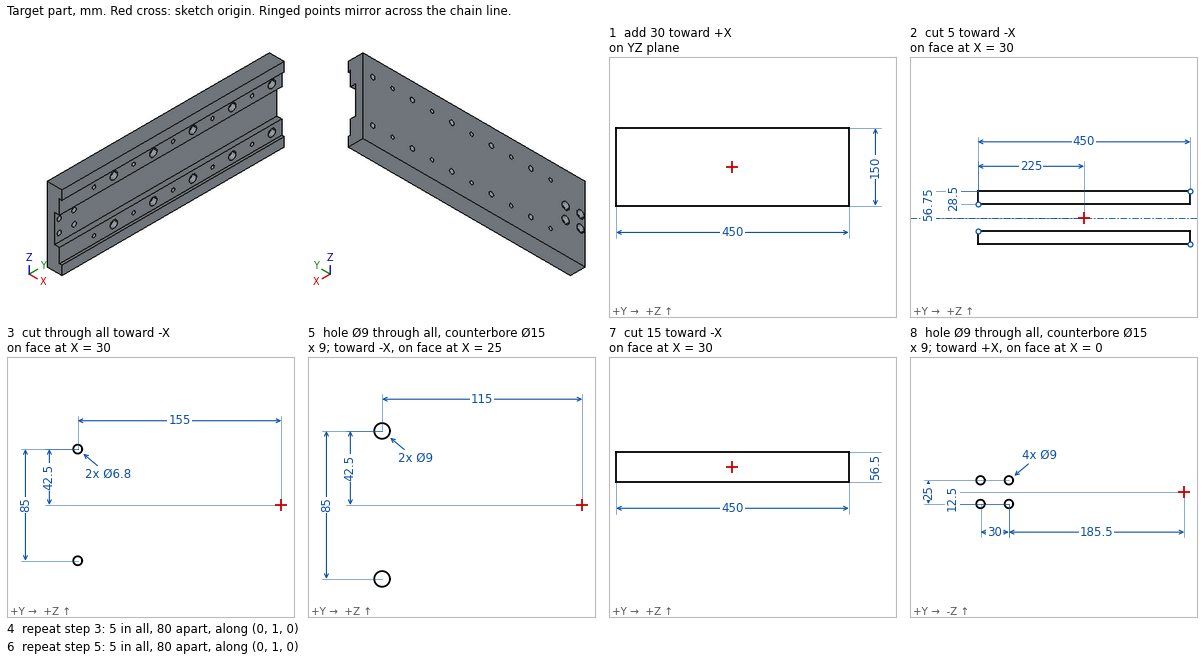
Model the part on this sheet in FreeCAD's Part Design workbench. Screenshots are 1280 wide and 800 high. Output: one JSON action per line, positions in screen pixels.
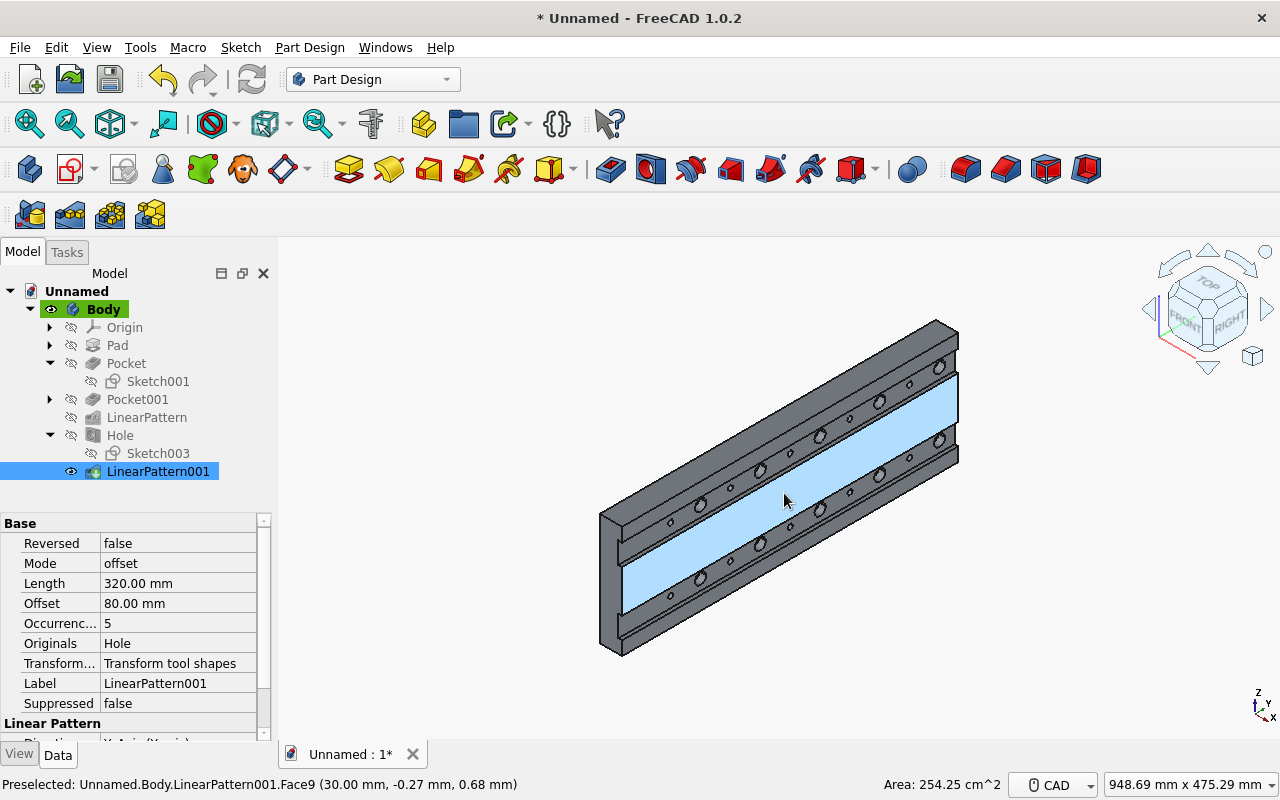
{"action": "left_click", "coordinate": [70, 170]}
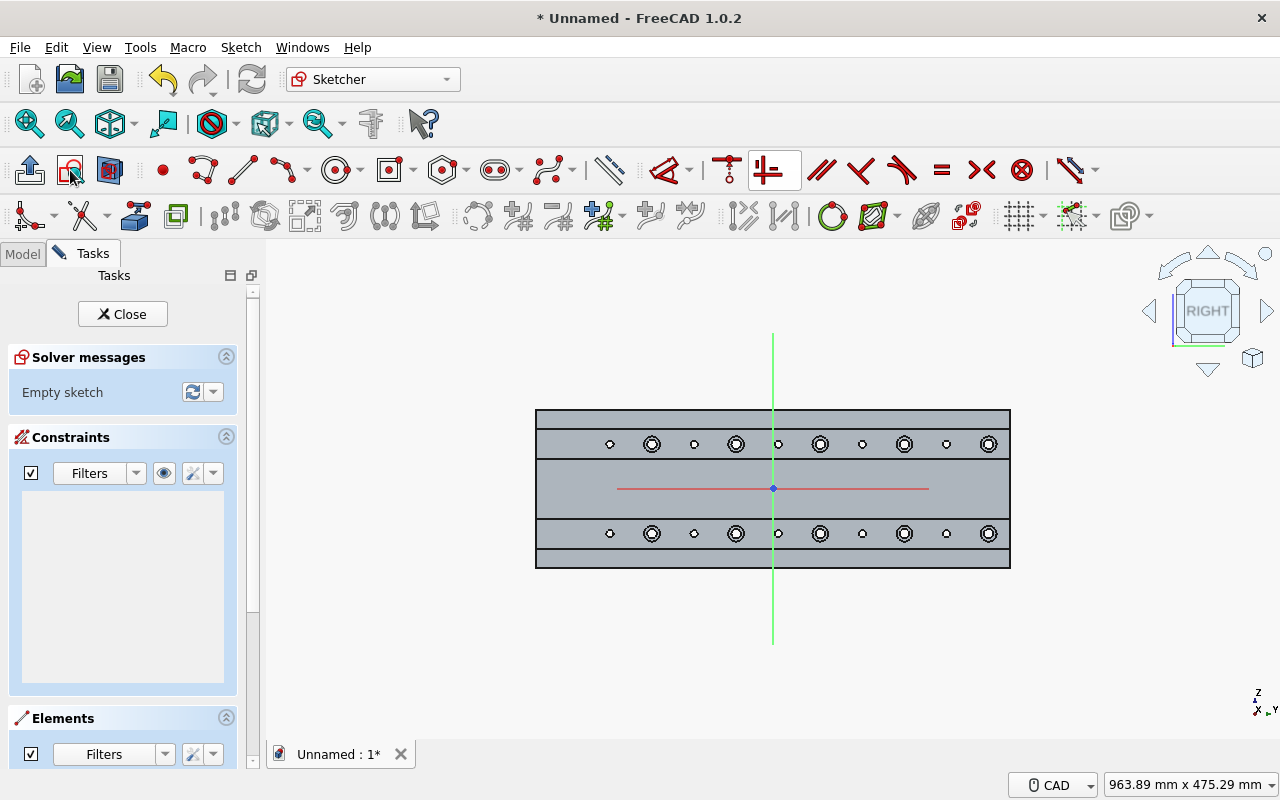
{"action": "left_click", "coordinate": [390, 170]}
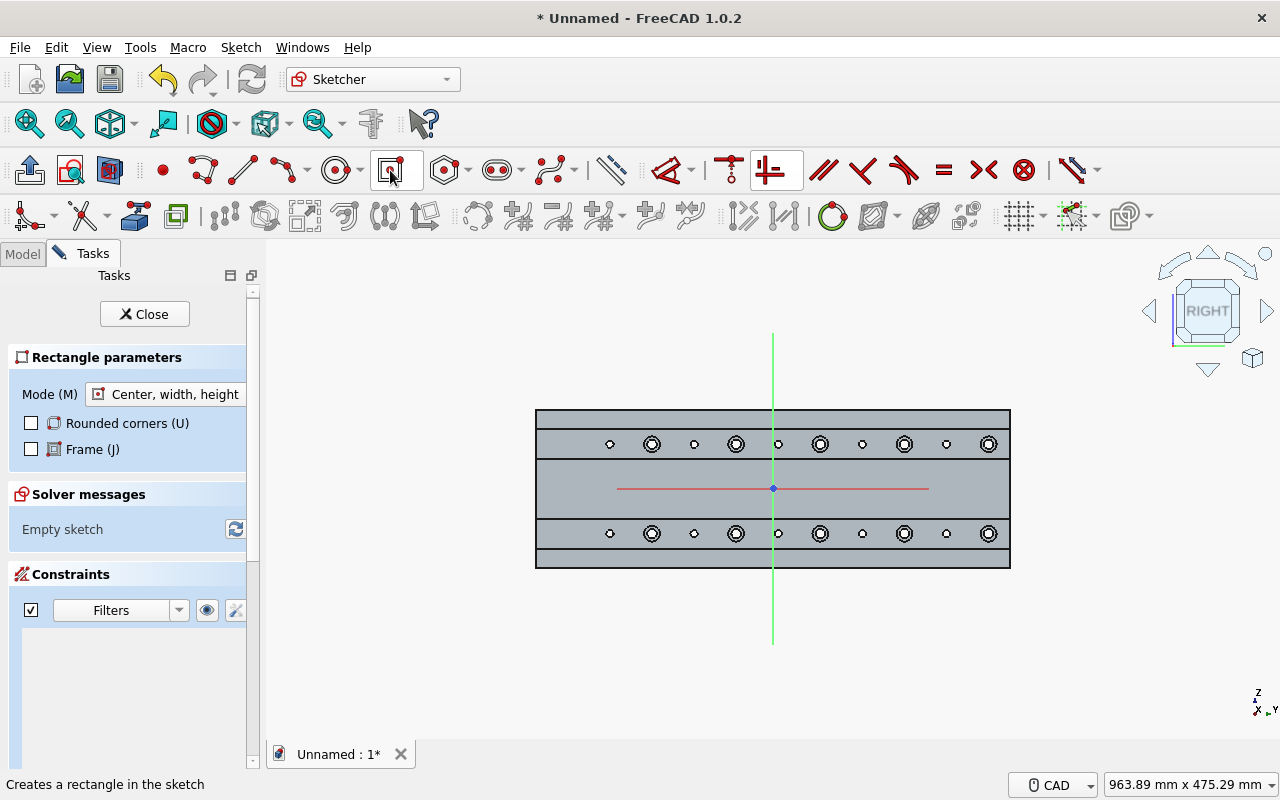
{"action": "left_click", "coordinate": [773, 489]}
{"action": "left_click", "coordinate": [1010, 459]}
{"action": "key", "text": "Escape"}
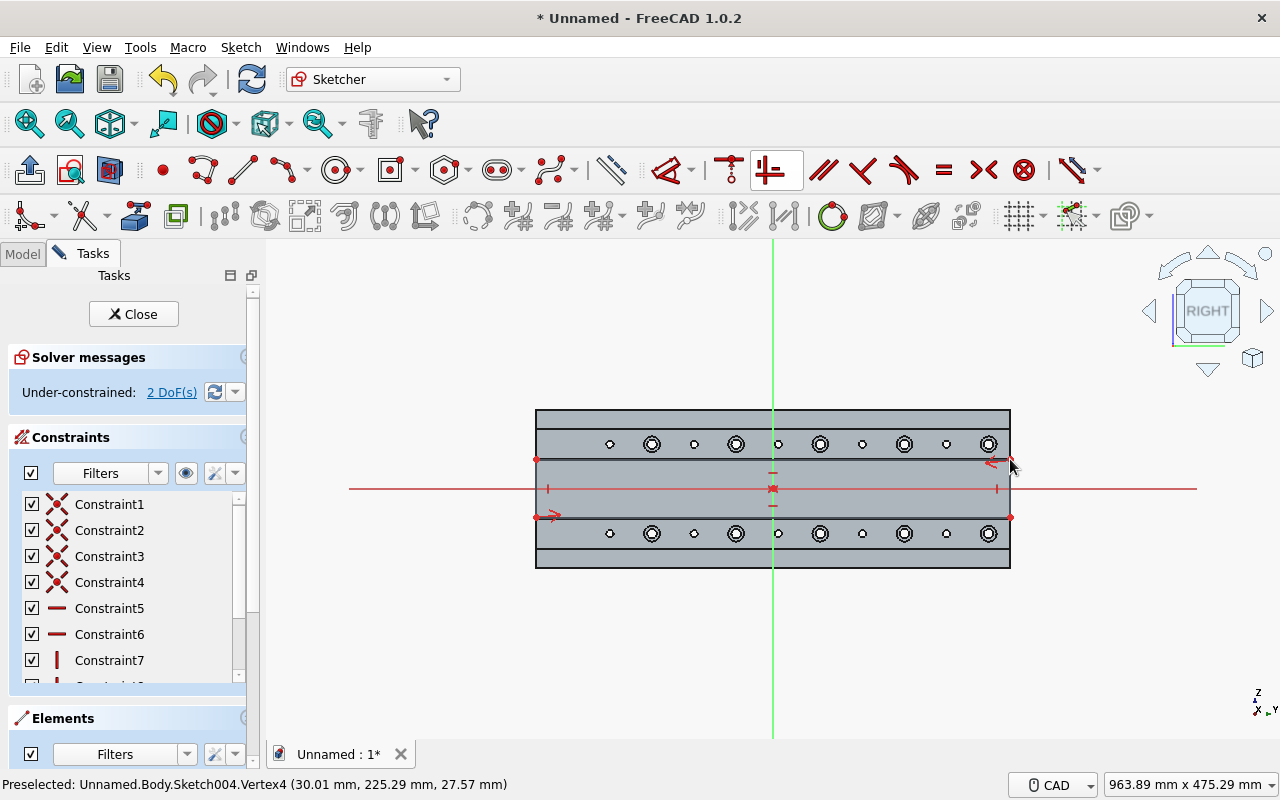
{"action": "left_click", "coordinate": [666, 170]}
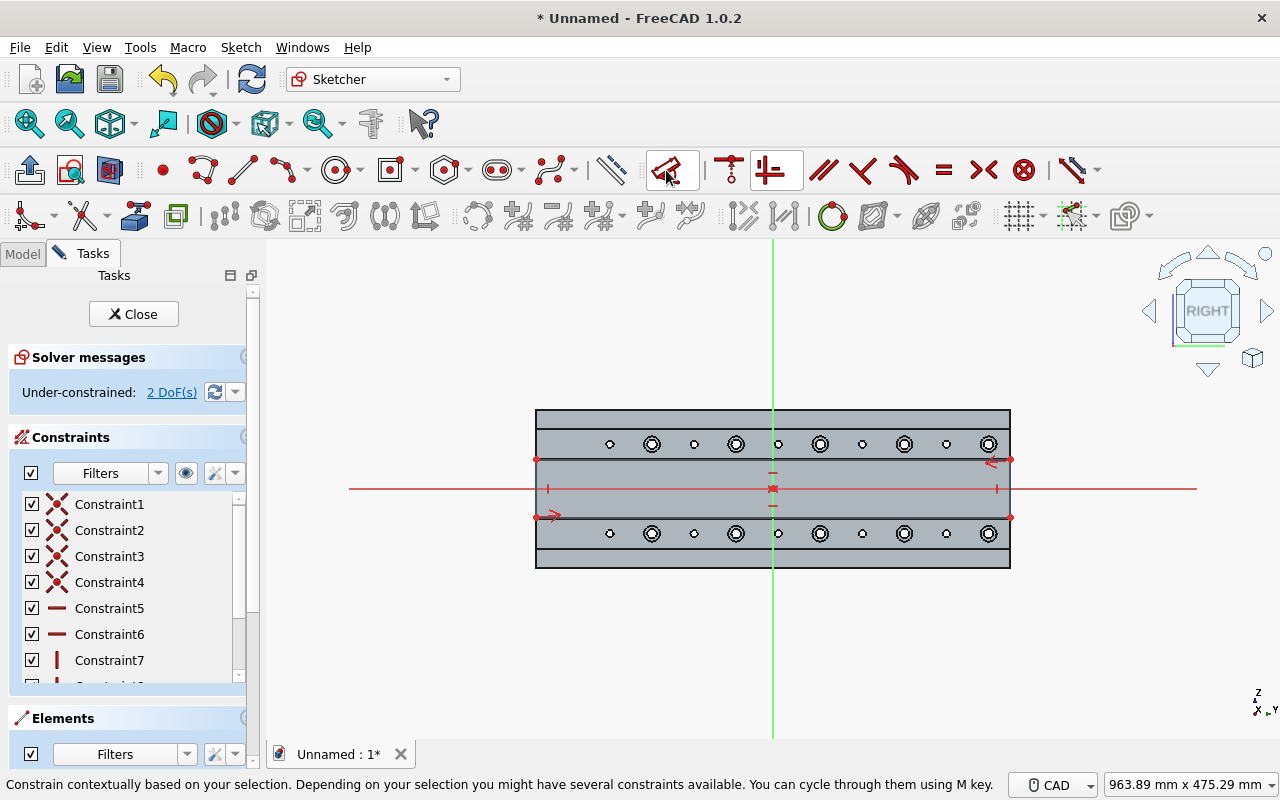
{"action": "left_click", "coordinate": [678, 518]}
{"action": "left_click", "coordinate": [664, 552]}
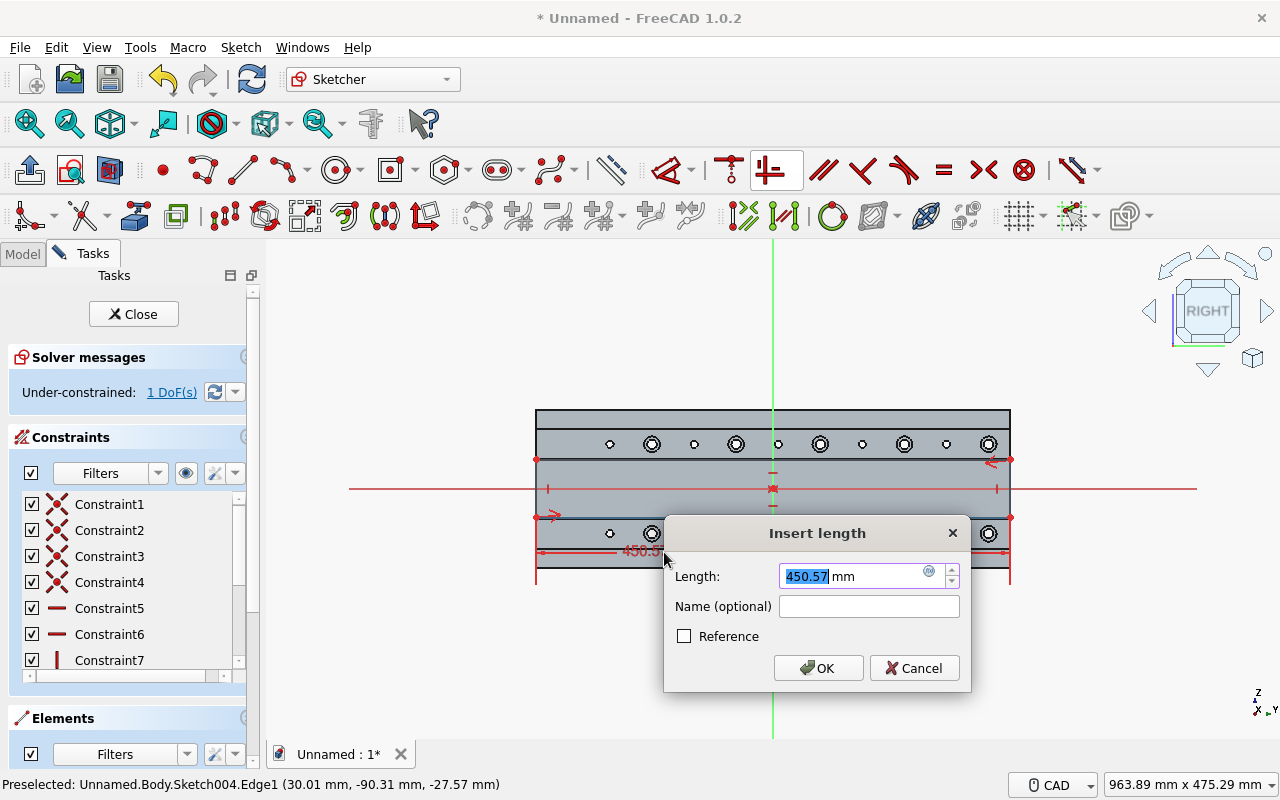
{"action": "type", "text": "450"}
{"action": "key", "text": "Return"}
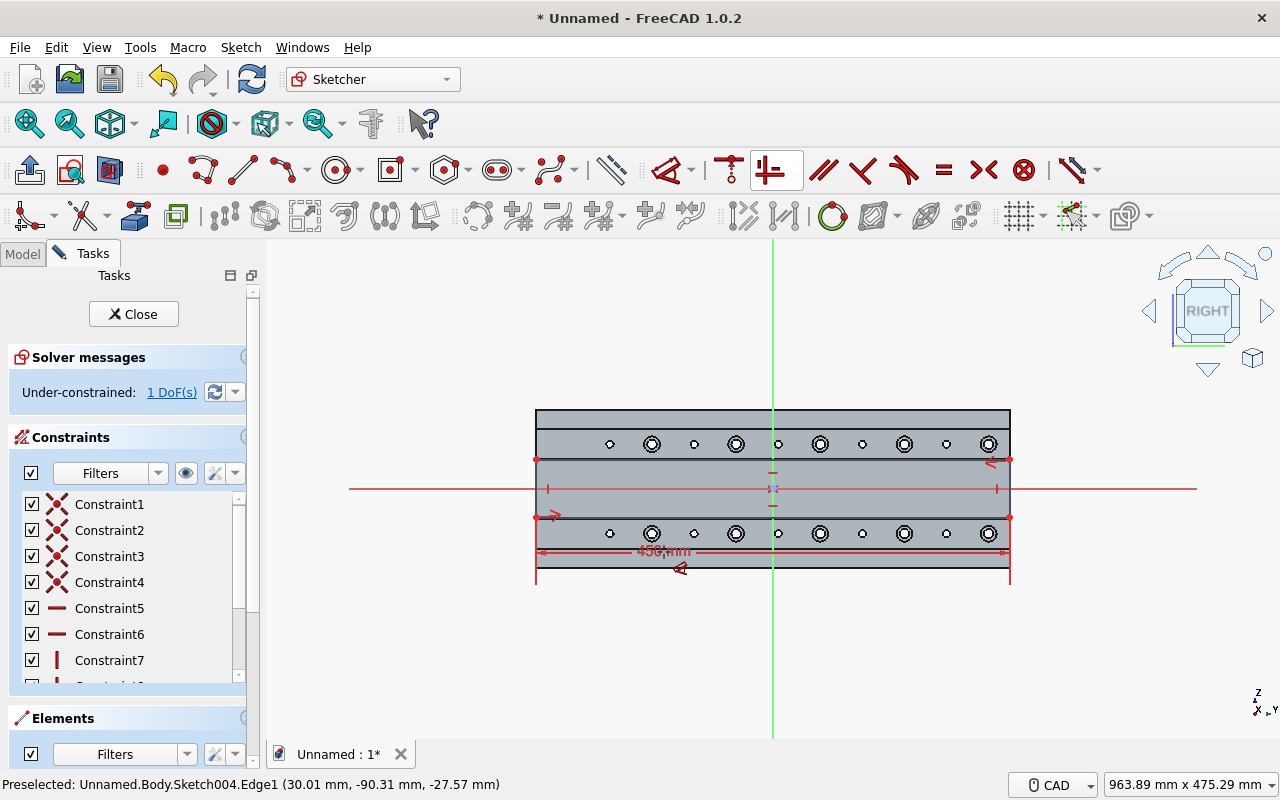
{"action": "left_click", "coordinate": [1010, 501]}
{"action": "left_click", "coordinate": [1044, 476]}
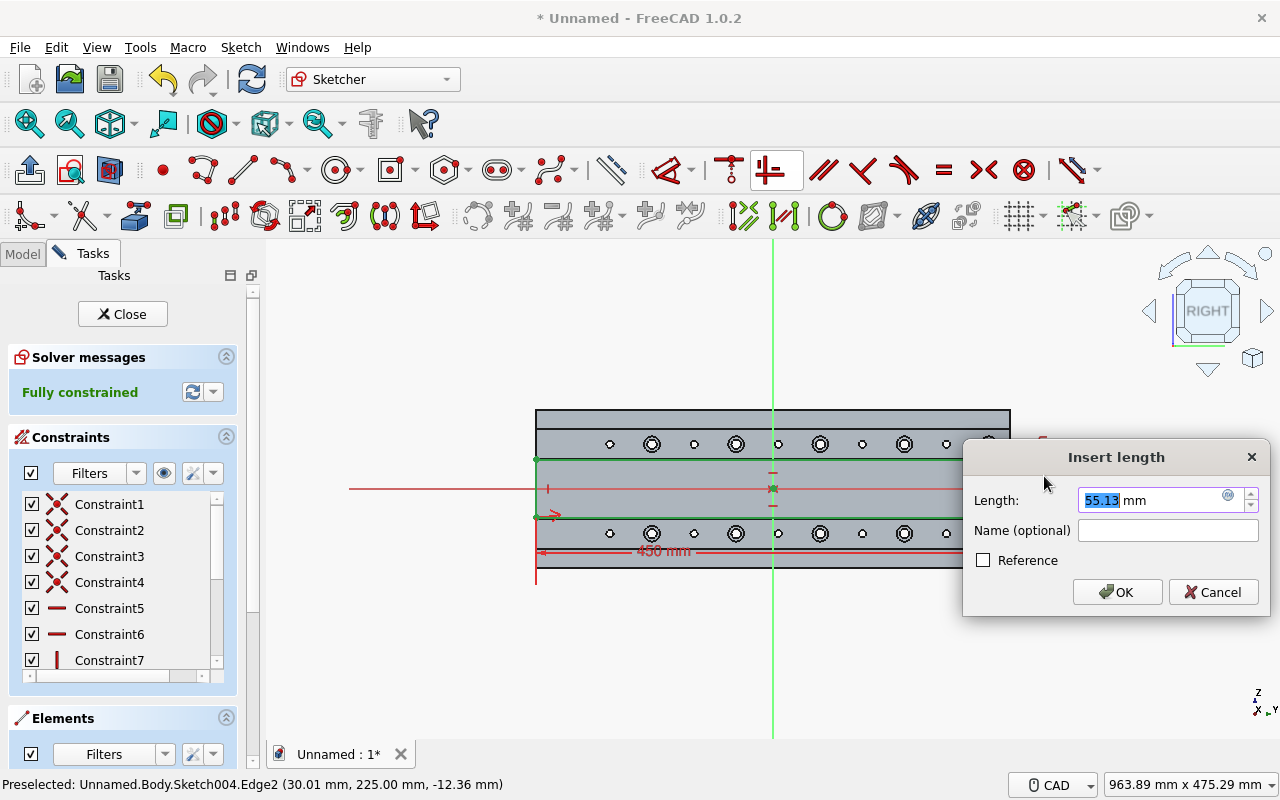
{"action": "type", "text": "56.5"}
{"action": "key", "text": "Return"}
{"action": "key", "text": "Escape"}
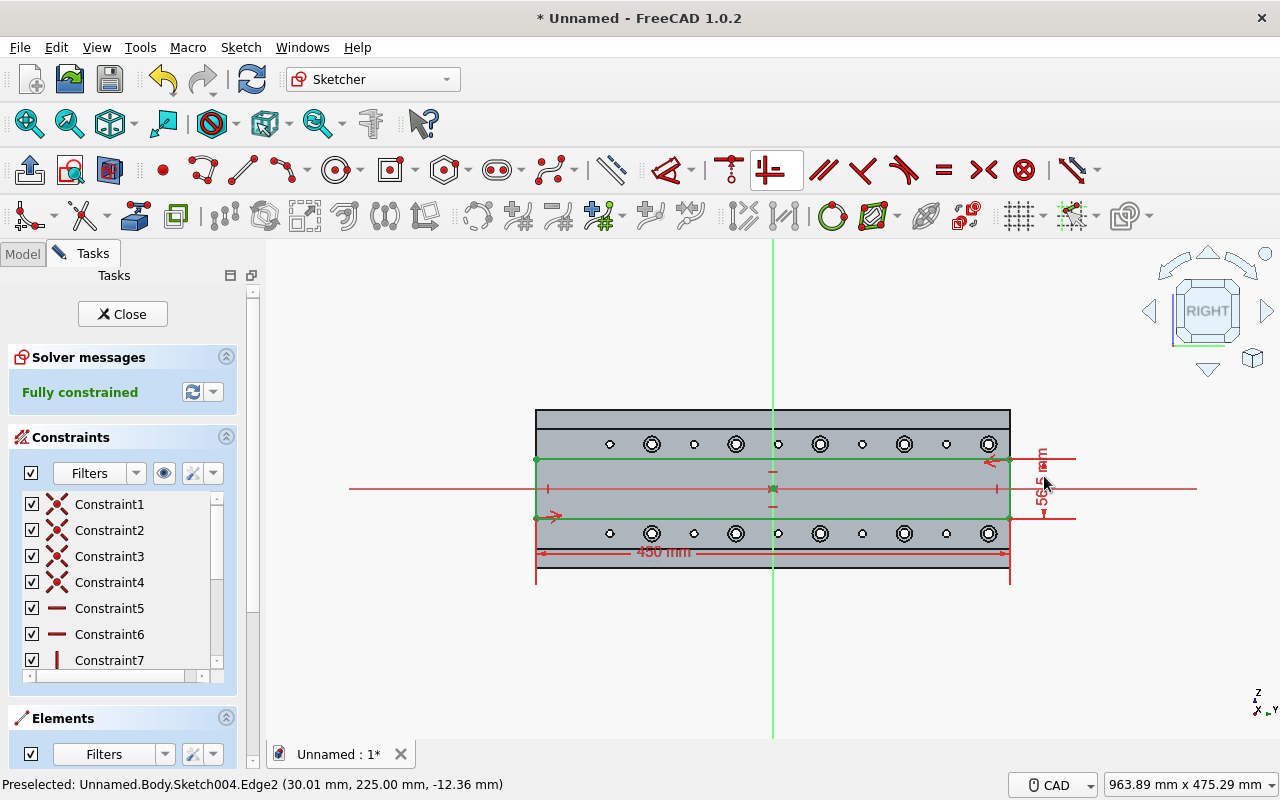
{"action": "left_click", "coordinate": [123, 314]}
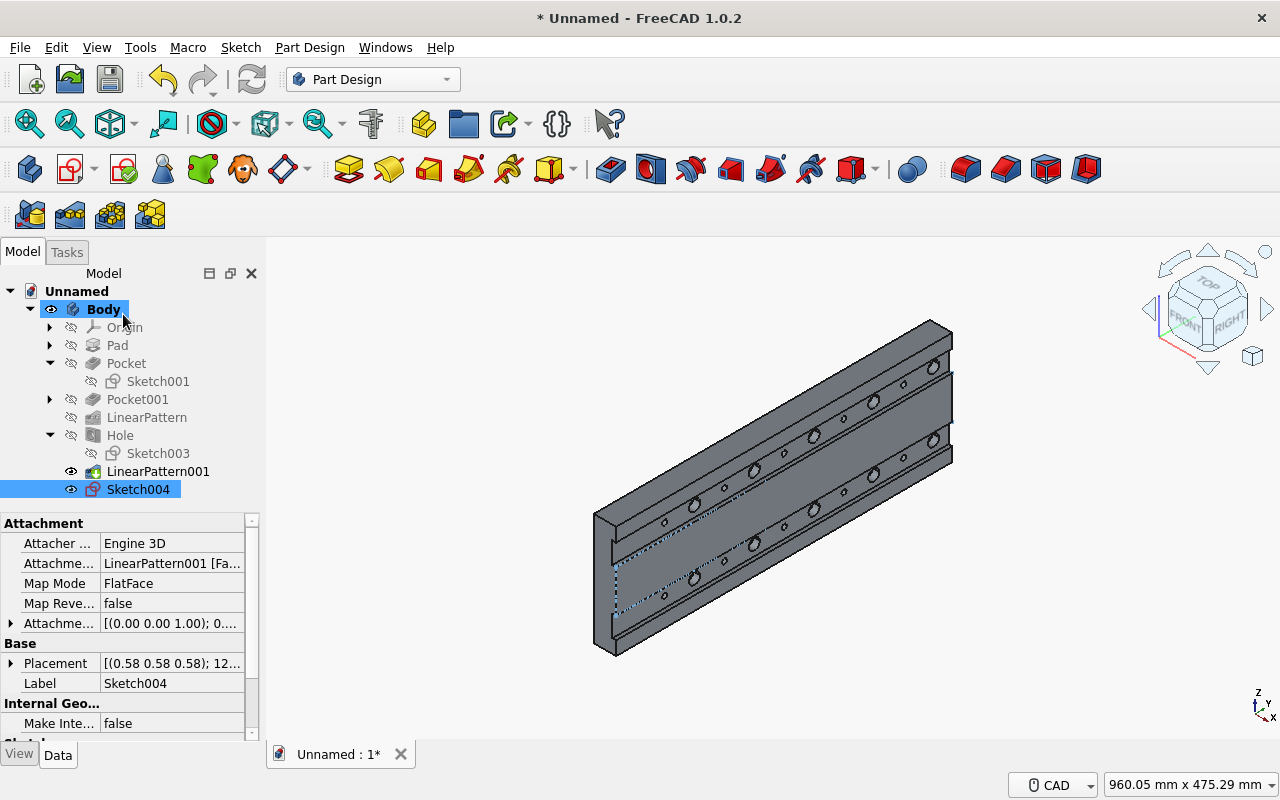
{"action": "left_click", "coordinate": [612, 170]}